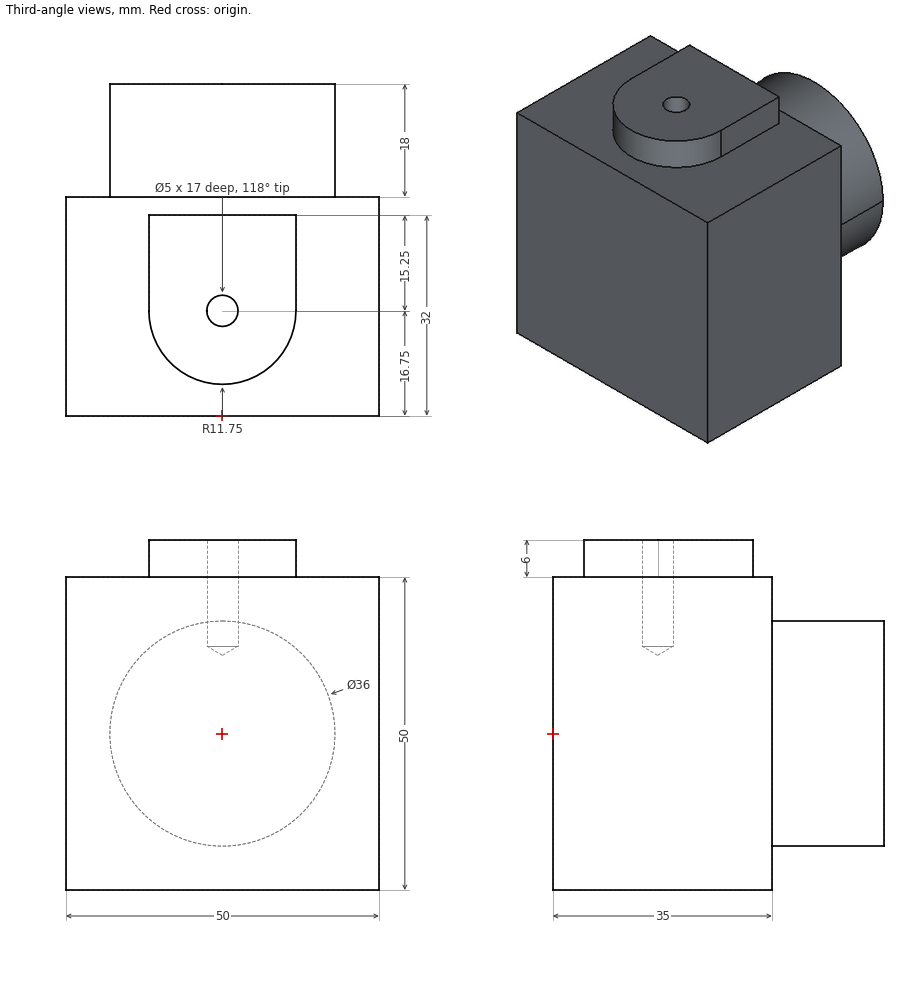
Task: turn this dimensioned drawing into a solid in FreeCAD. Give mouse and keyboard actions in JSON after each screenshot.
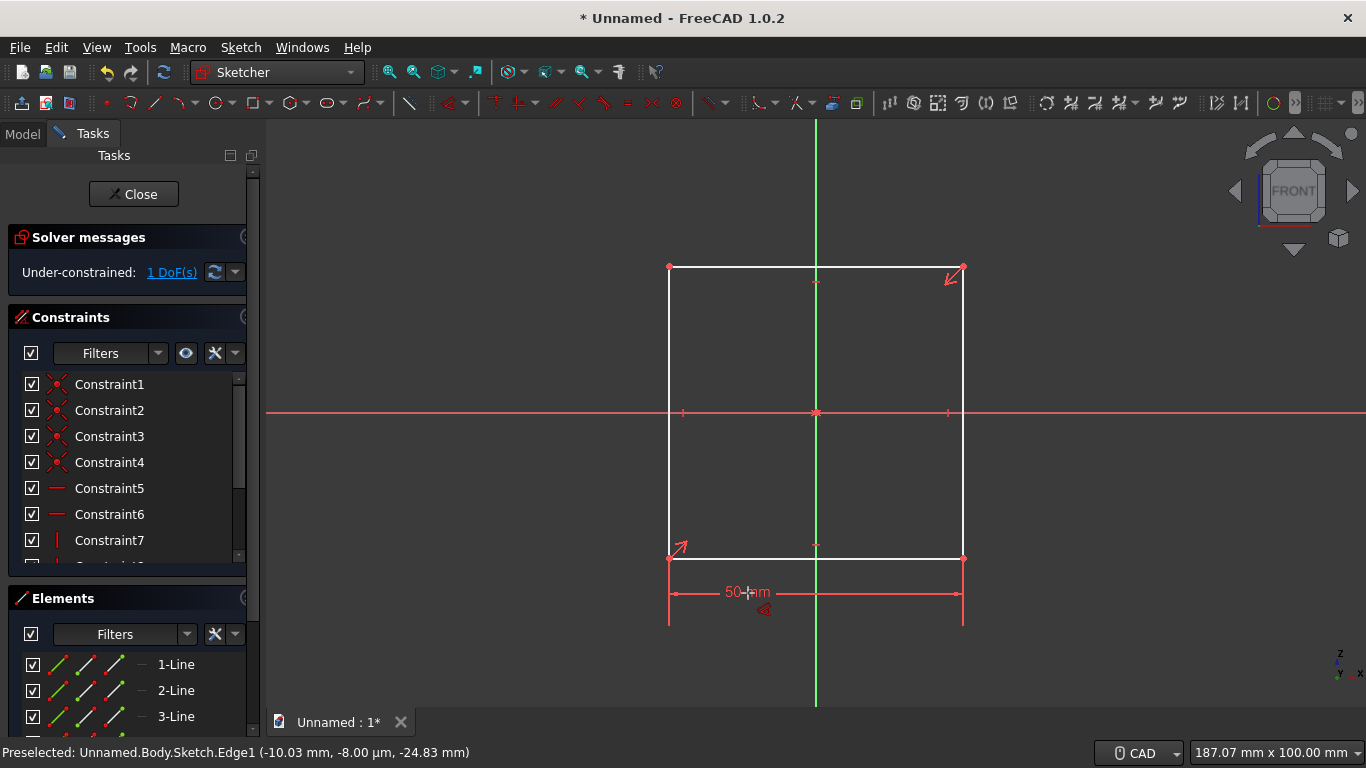
{"action": "left_click", "coordinate": [963, 471]}
{"action": "left_click", "coordinate": [997, 346]}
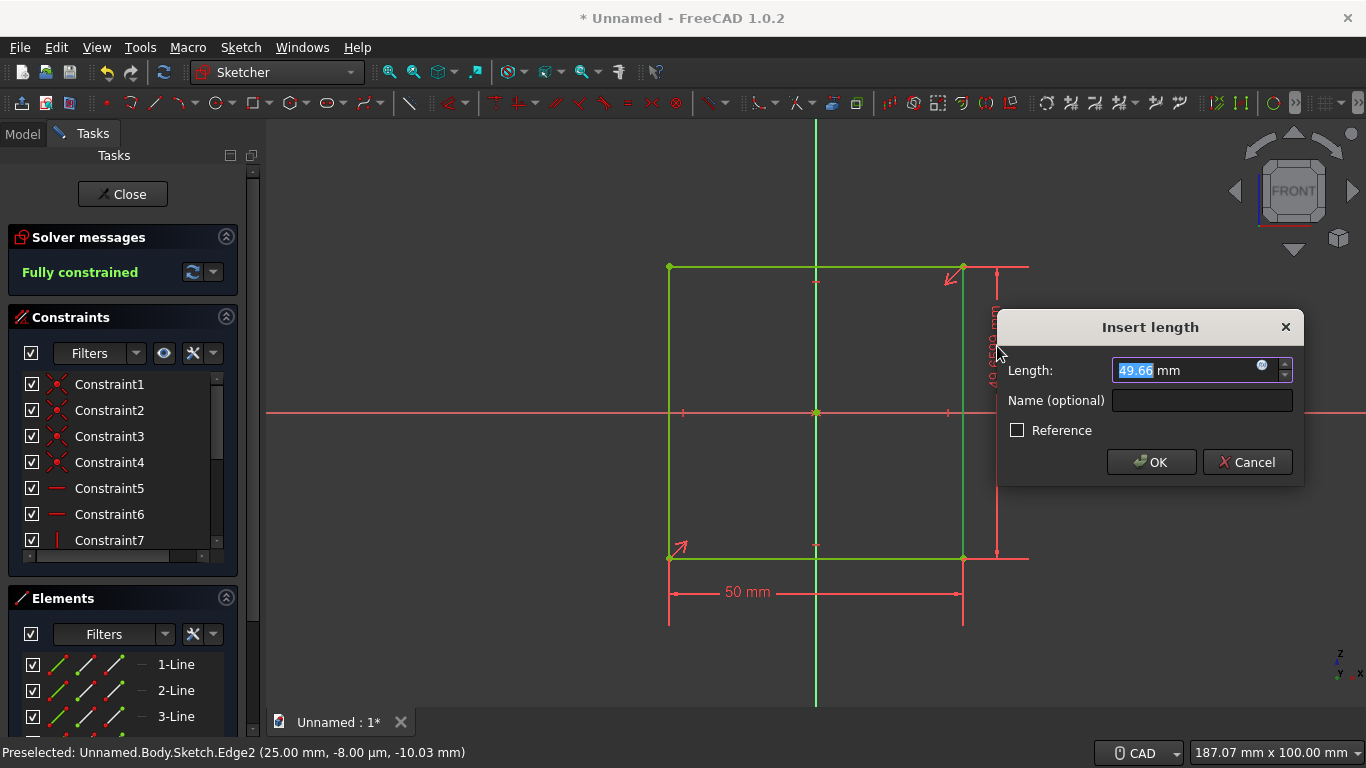
{"action": "type", "text": "50"}
{"action": "key", "text": "Return"}
{"action": "key", "text": "Escape"}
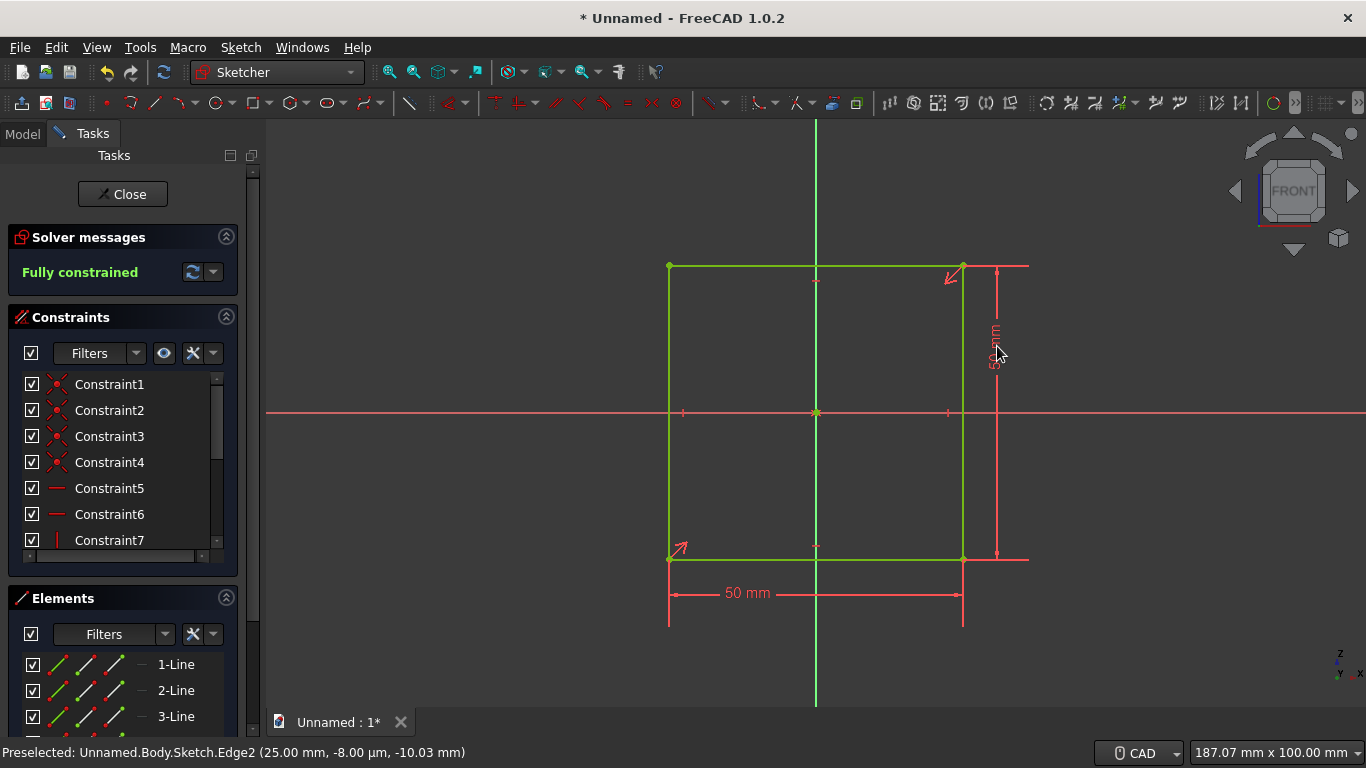
{"action": "left_click", "coordinate": [123, 194]}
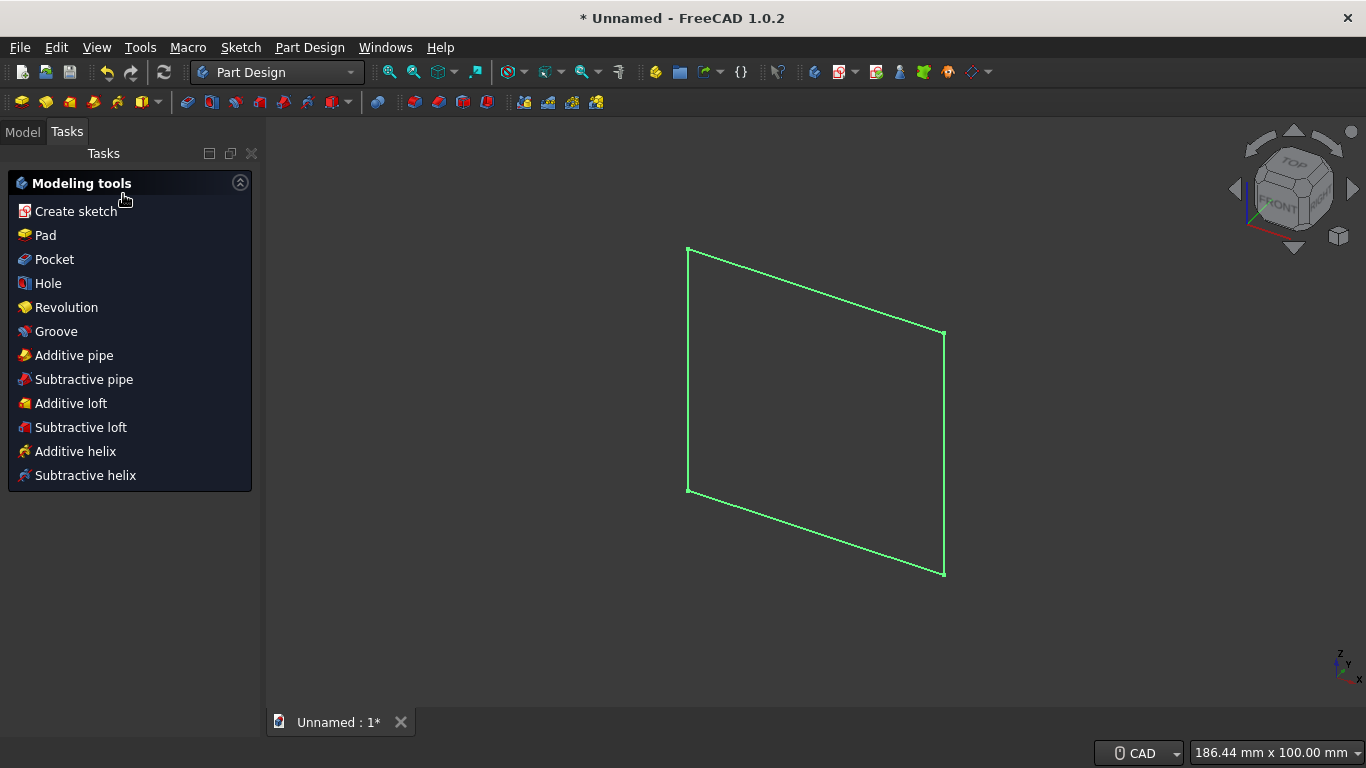
{"action": "left_click", "coordinate": [22, 102]}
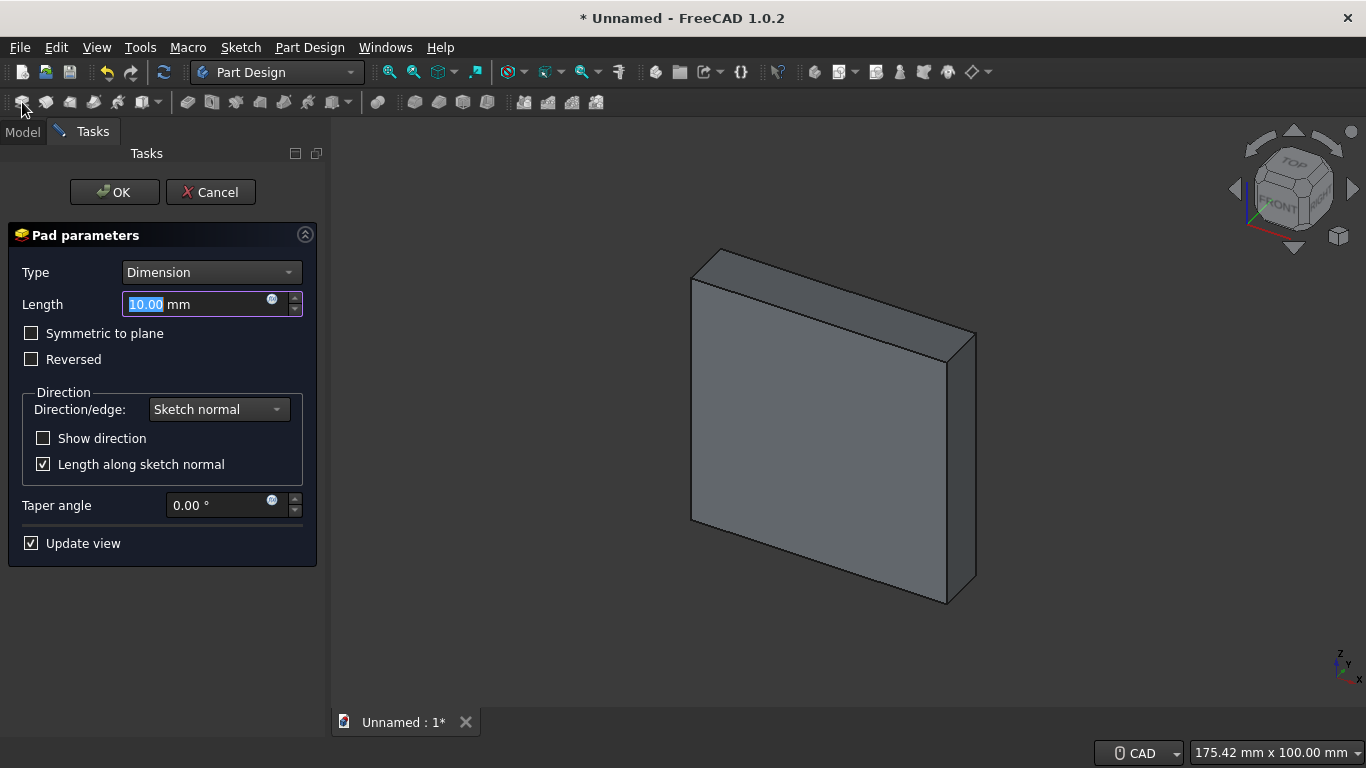
{"action": "type", "text": "35"}
{"action": "key", "text": "Tab"}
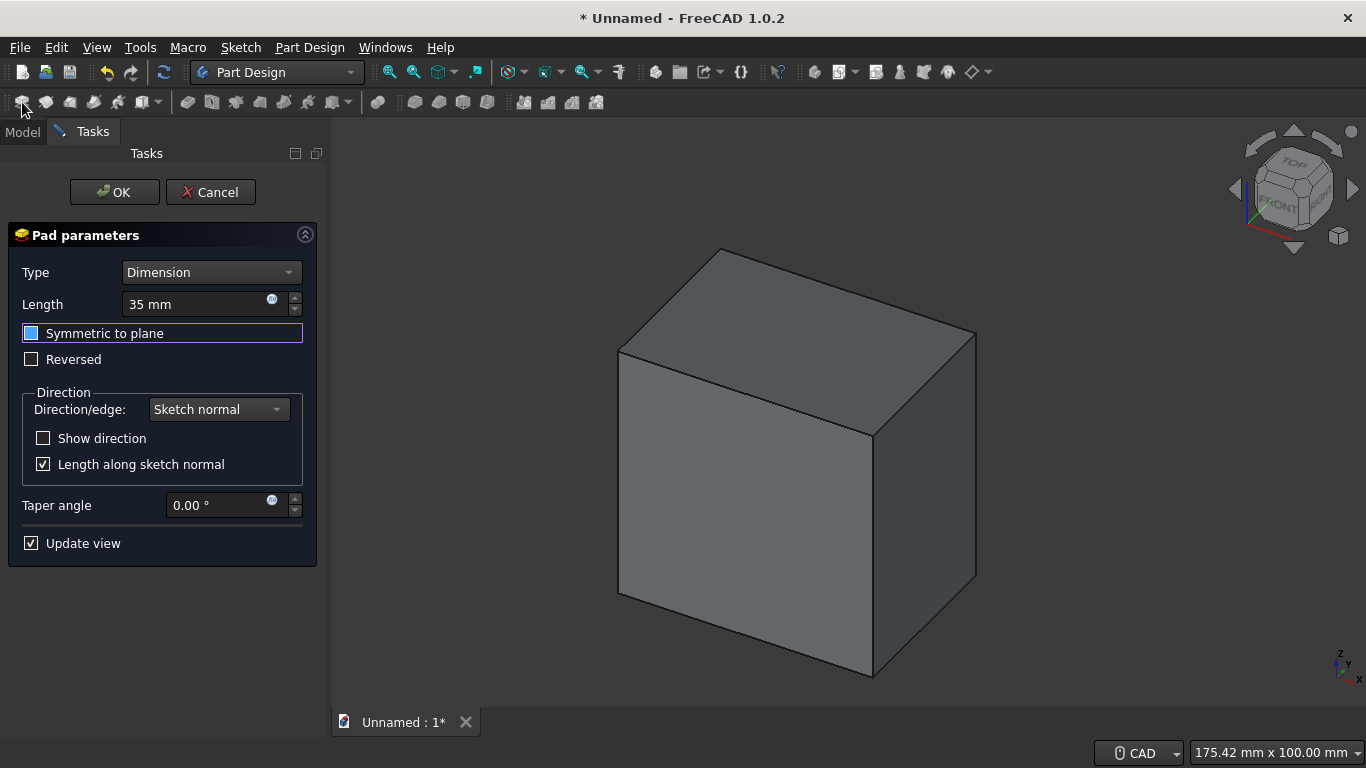
{"action": "left_click", "coordinate": [30, 359]}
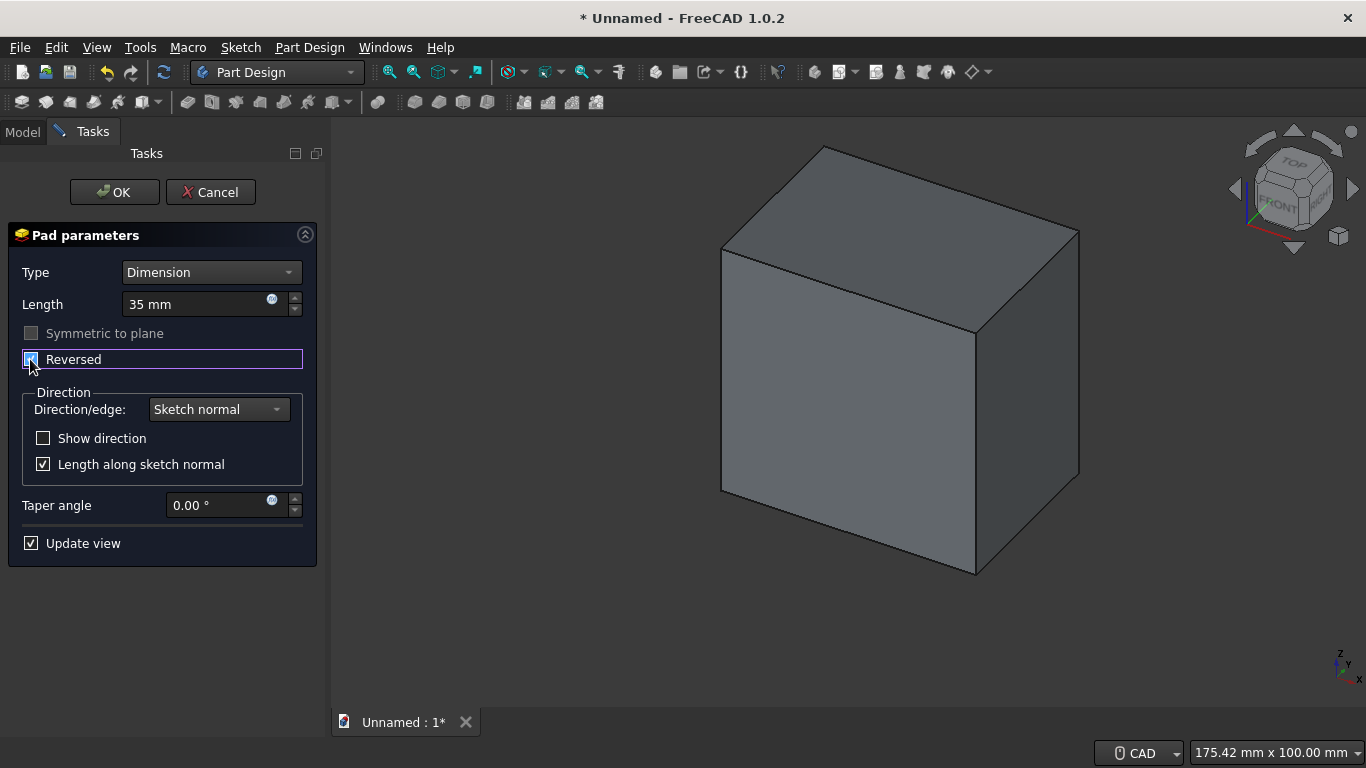
{"action": "left_click", "coordinate": [115, 192]}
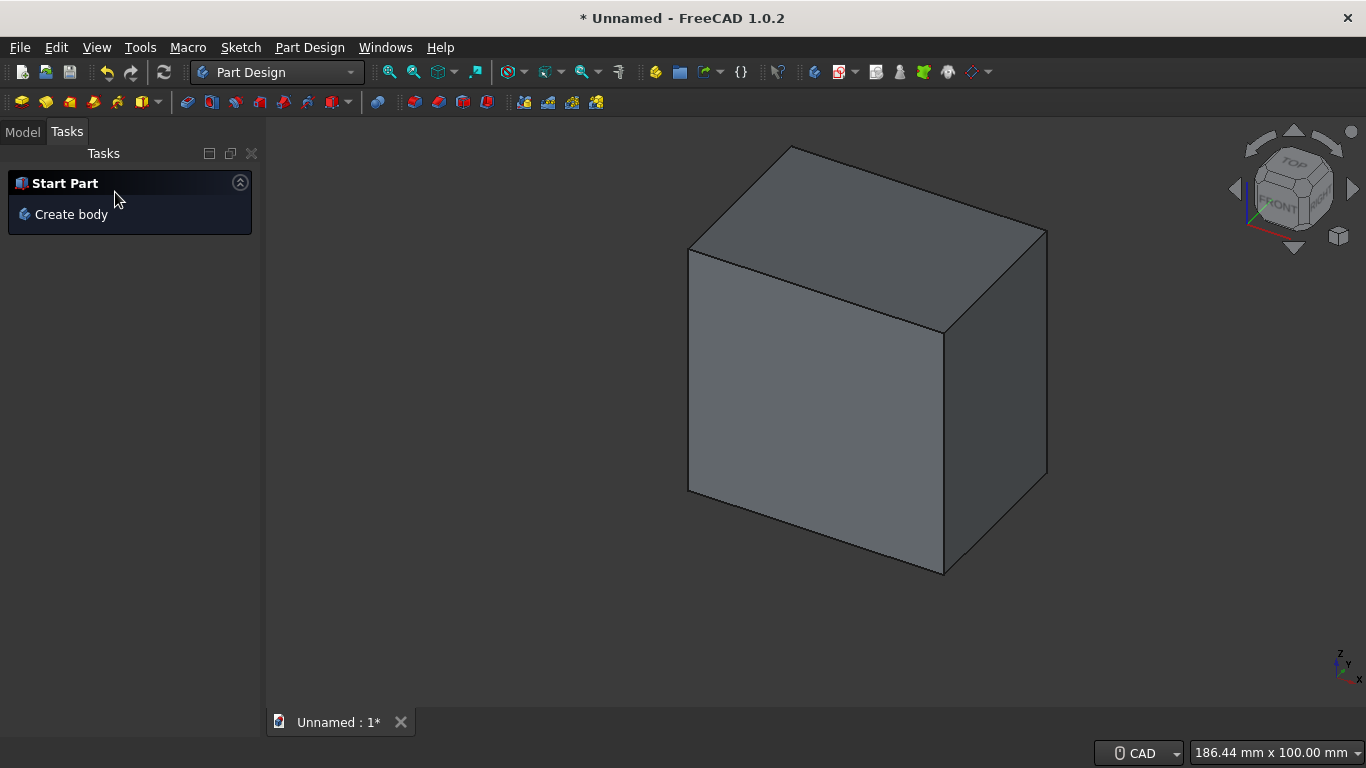
{"action": "key", "text": "4"}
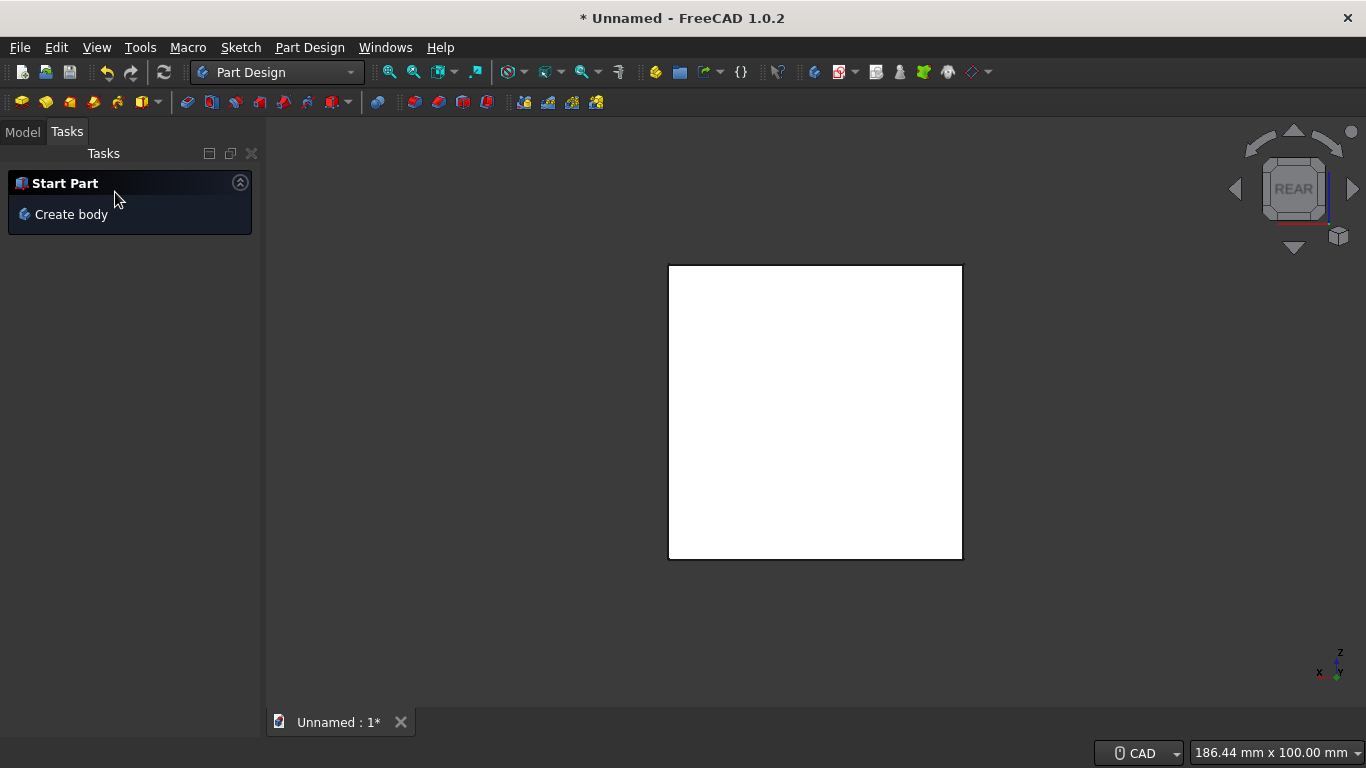
{"action": "left_click", "coordinate": [816, 411]}